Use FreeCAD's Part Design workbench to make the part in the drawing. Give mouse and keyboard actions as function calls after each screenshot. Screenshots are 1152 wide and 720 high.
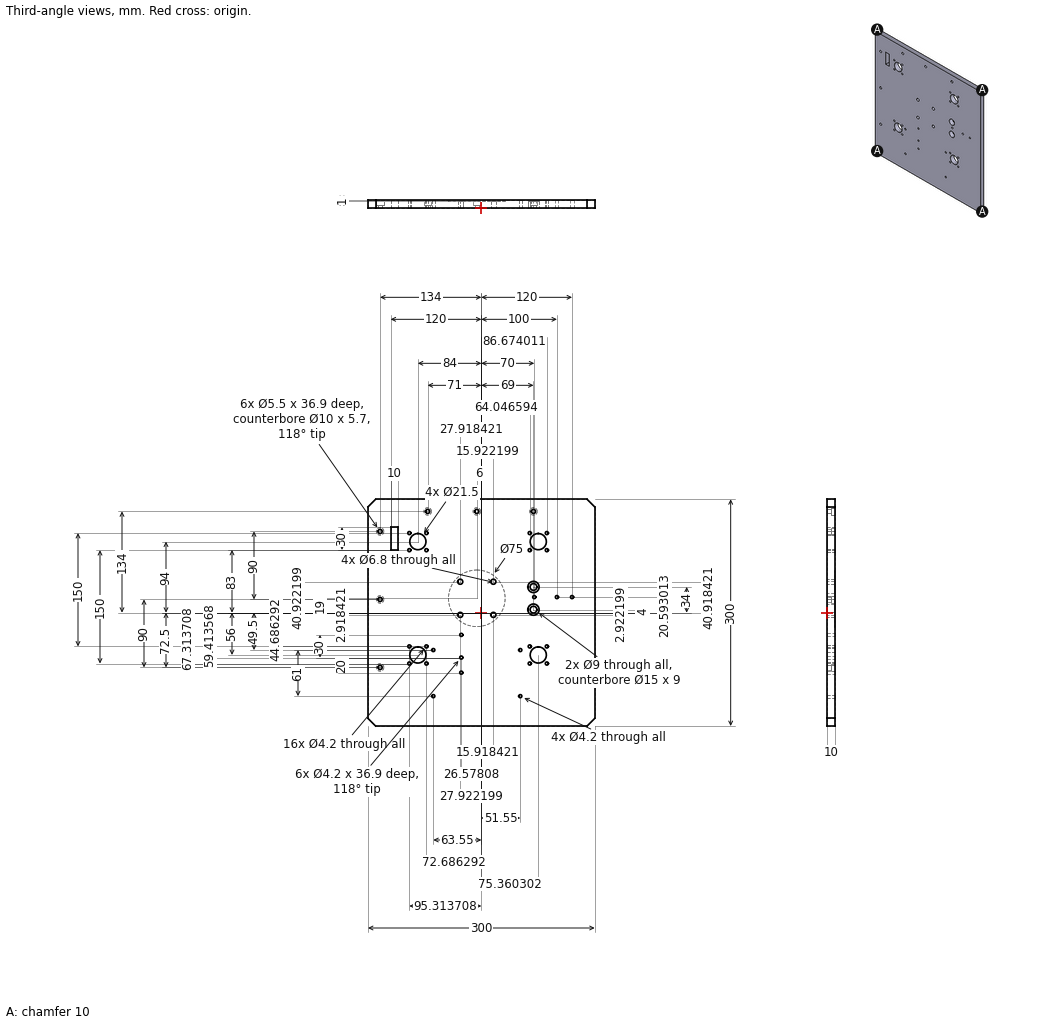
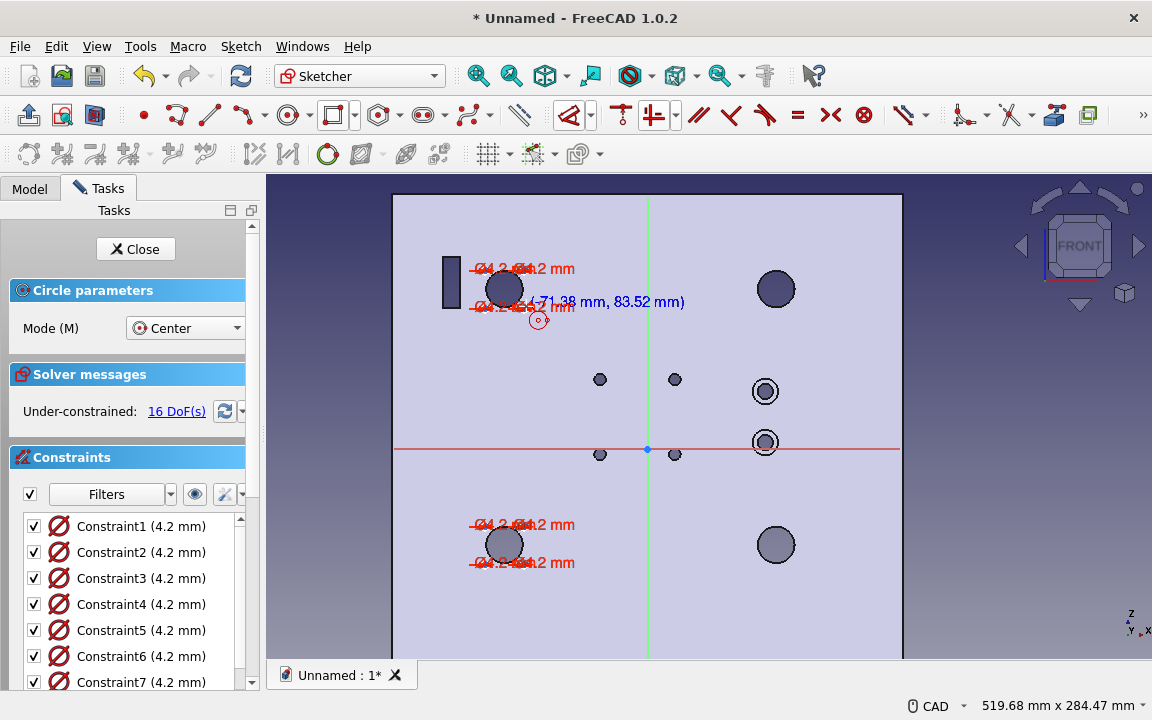
scroll(757, 308, up, 10)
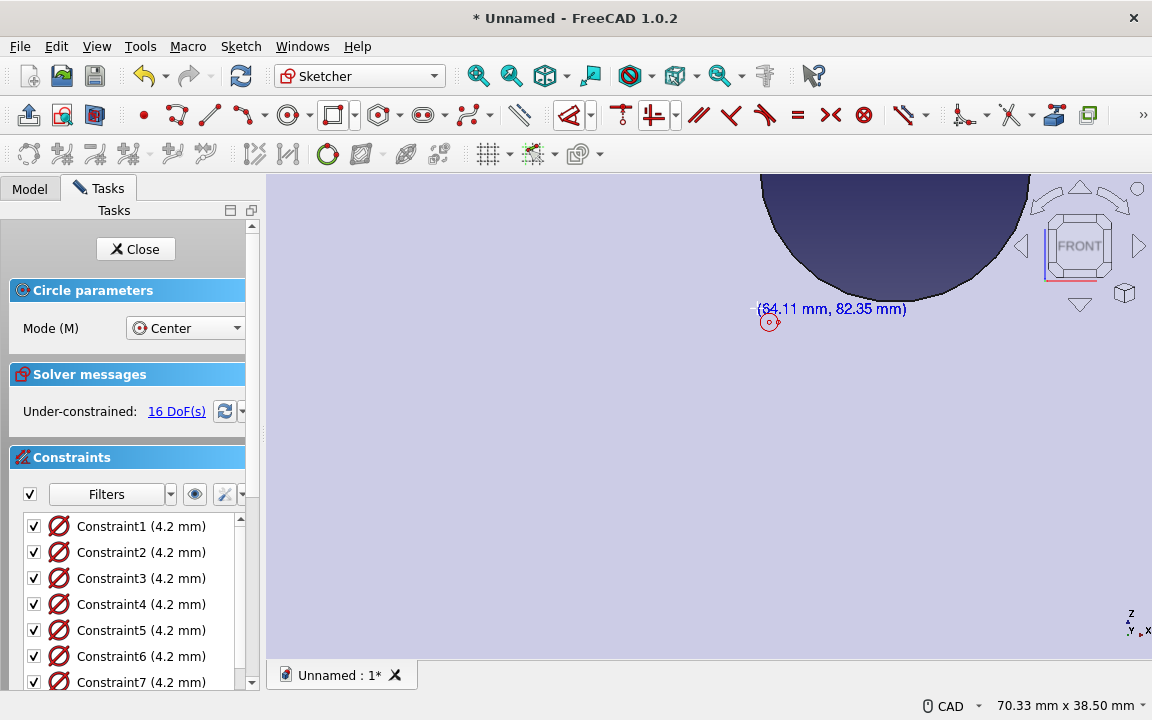
scroll(758, 308, down, 10)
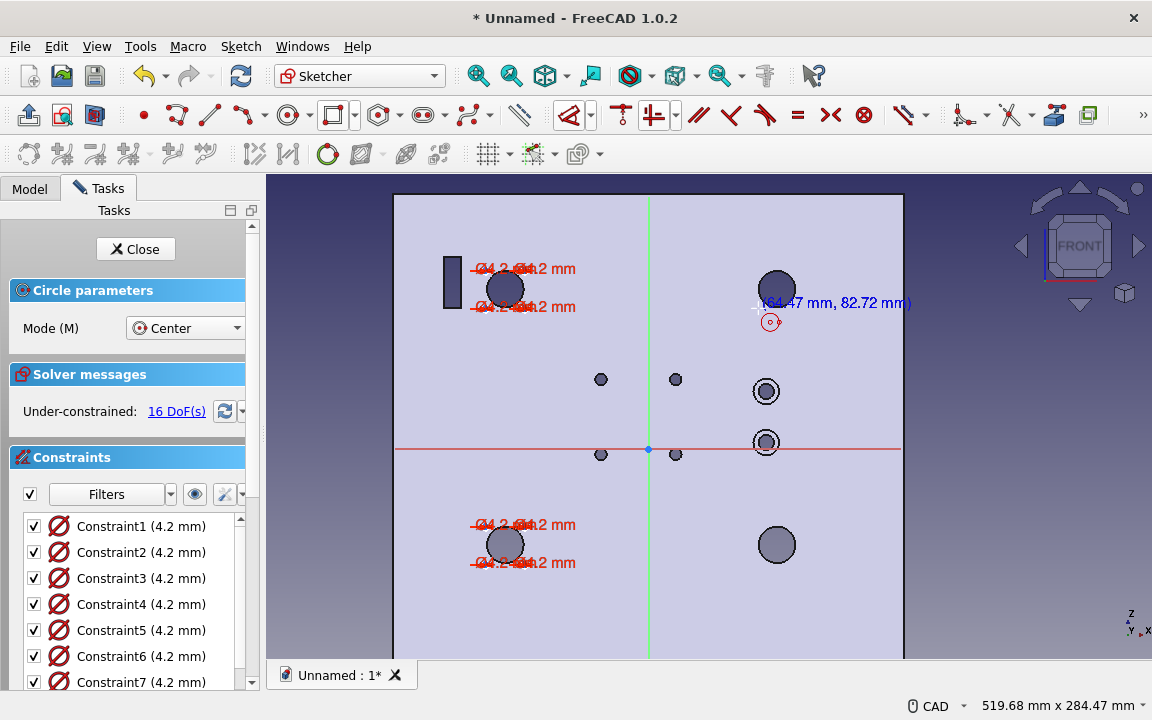
click(758, 308)
move(760, 306)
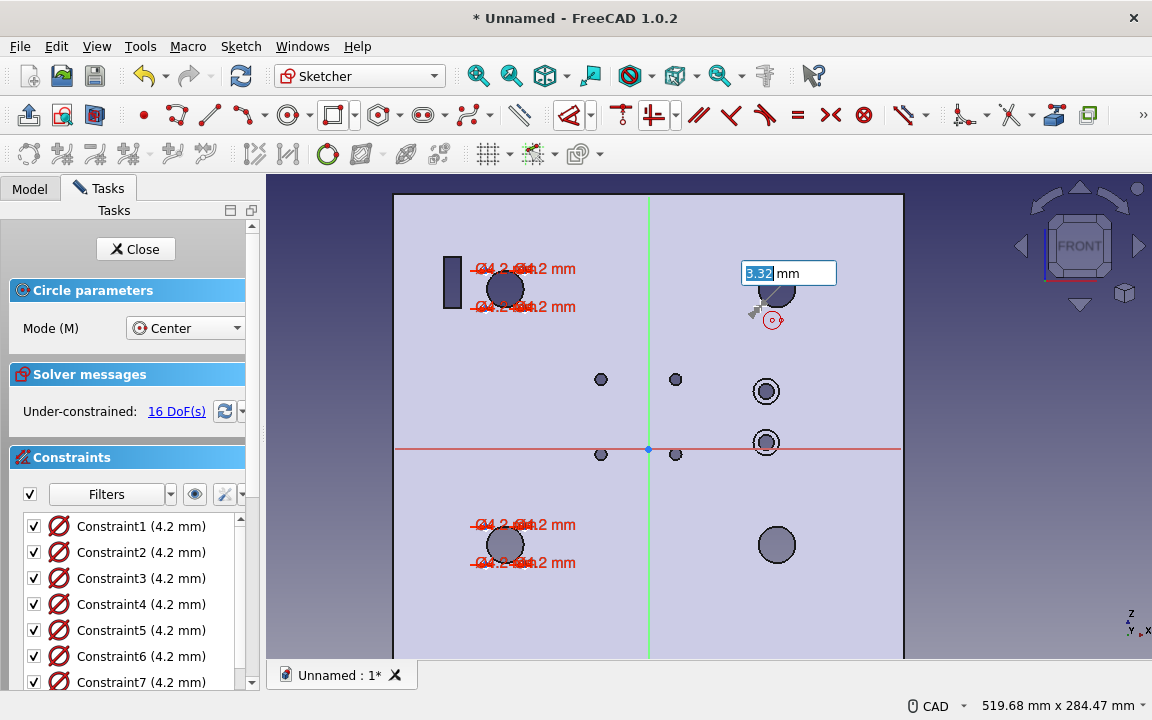
text(4.2)
key(Return)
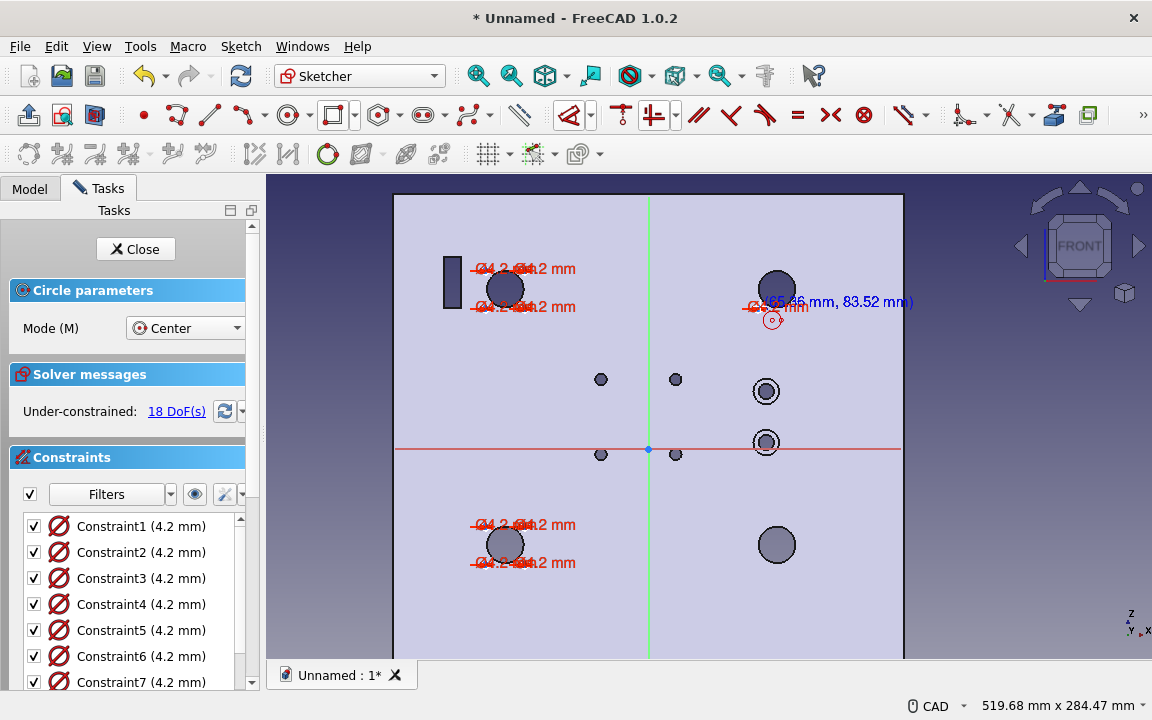
scroll(758, 270, up, 10)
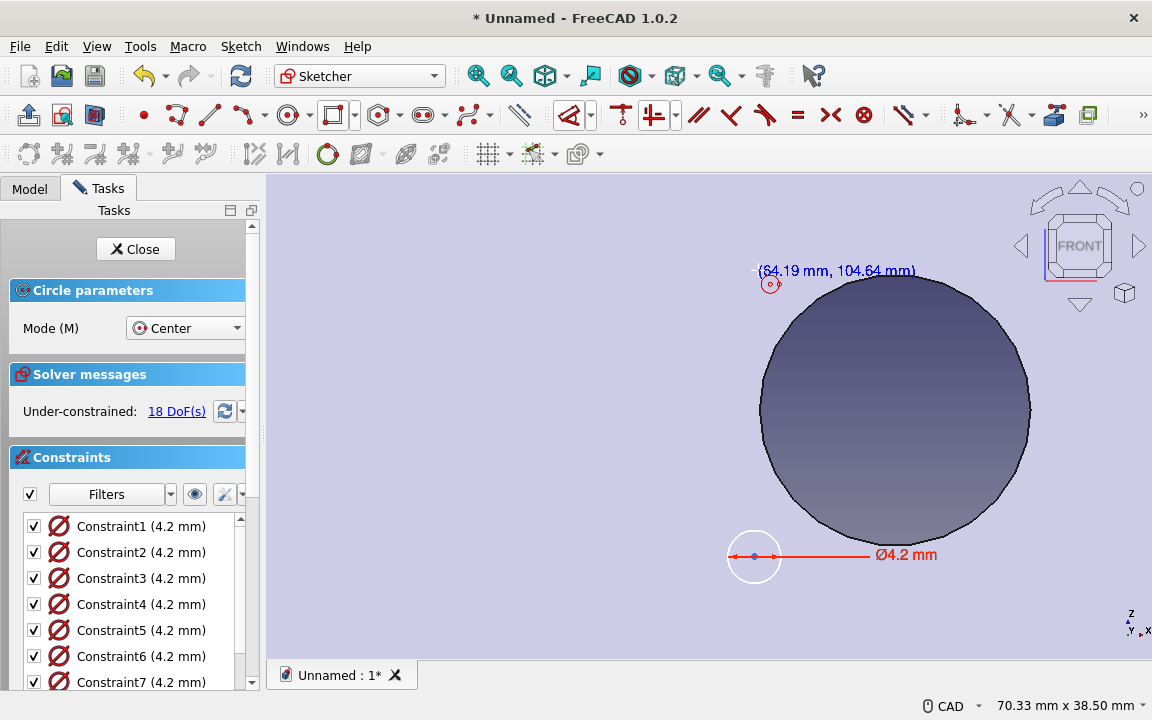
scroll(758, 270, down, 10)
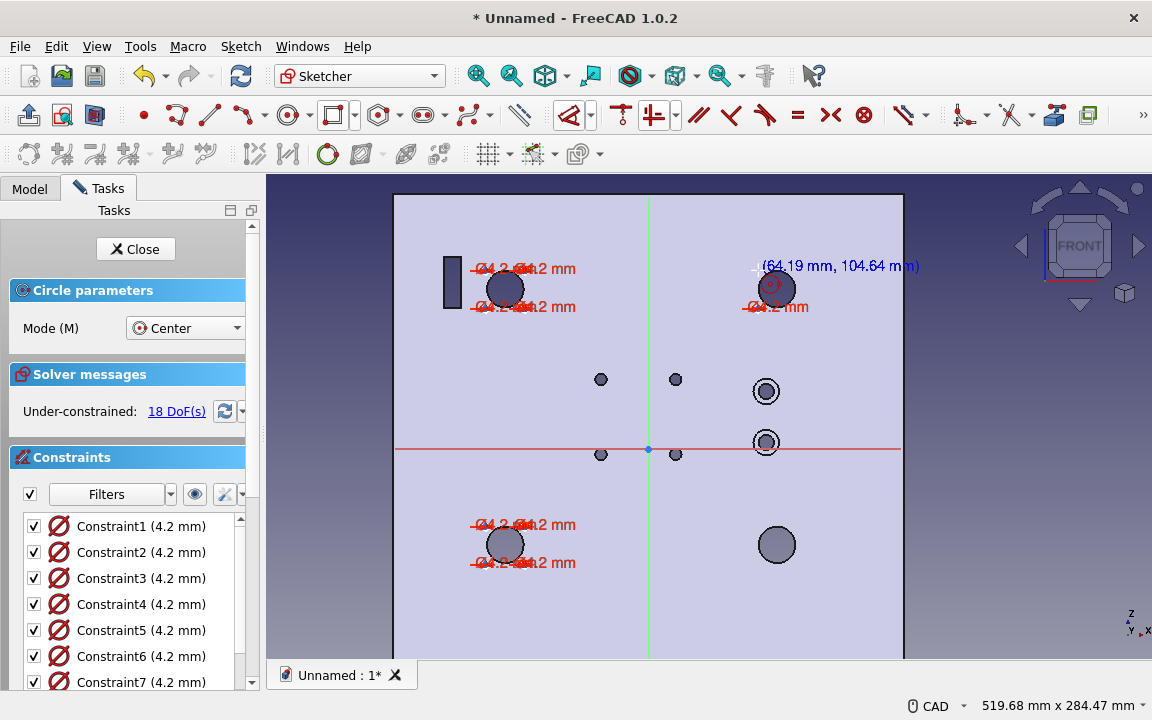
click(758, 270)
move(760, 267)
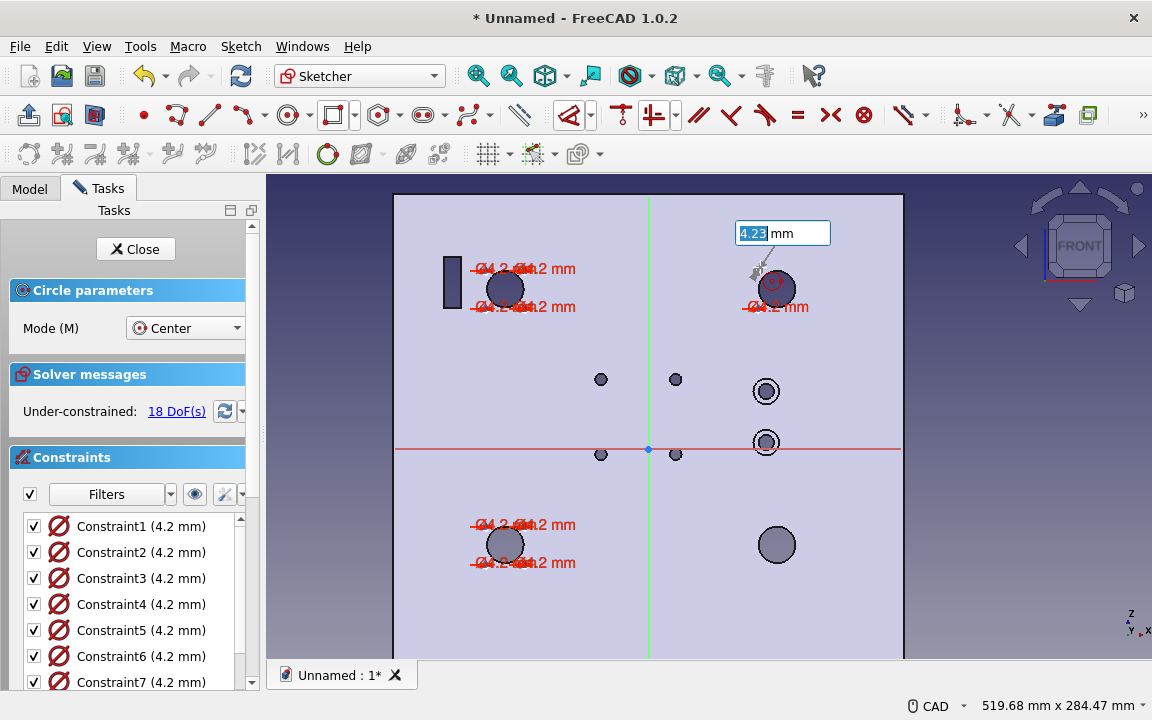
text(4.2)
key(Return)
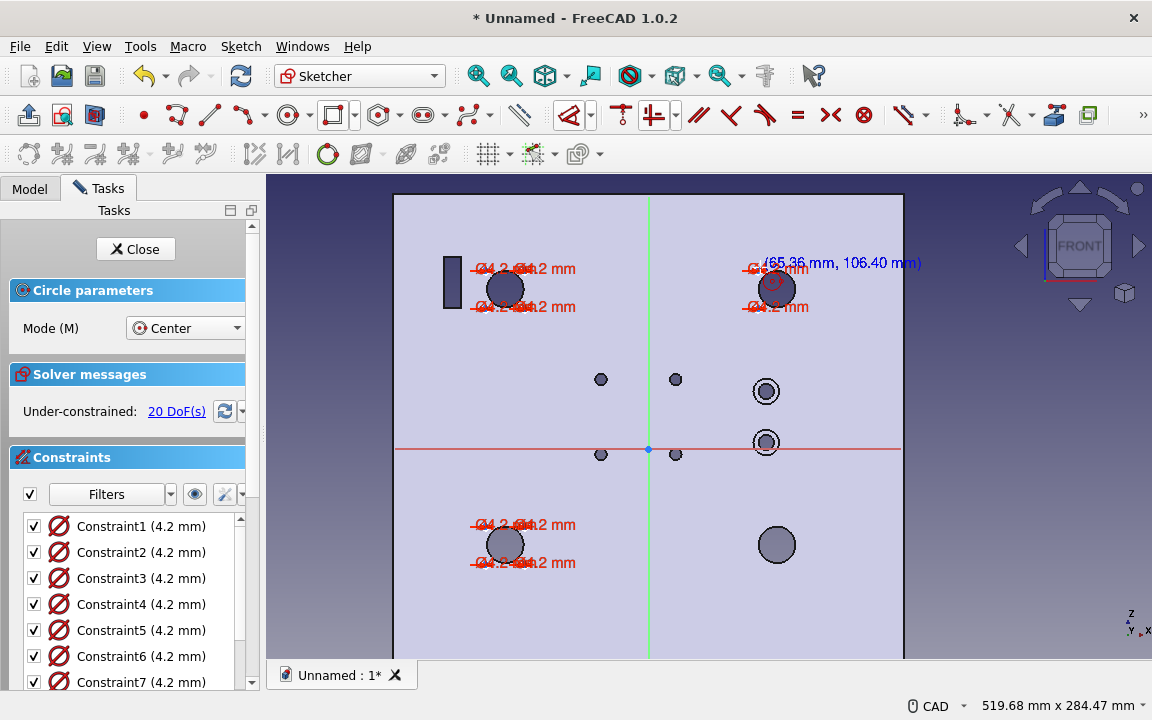
scroll(796, 270, up, 10)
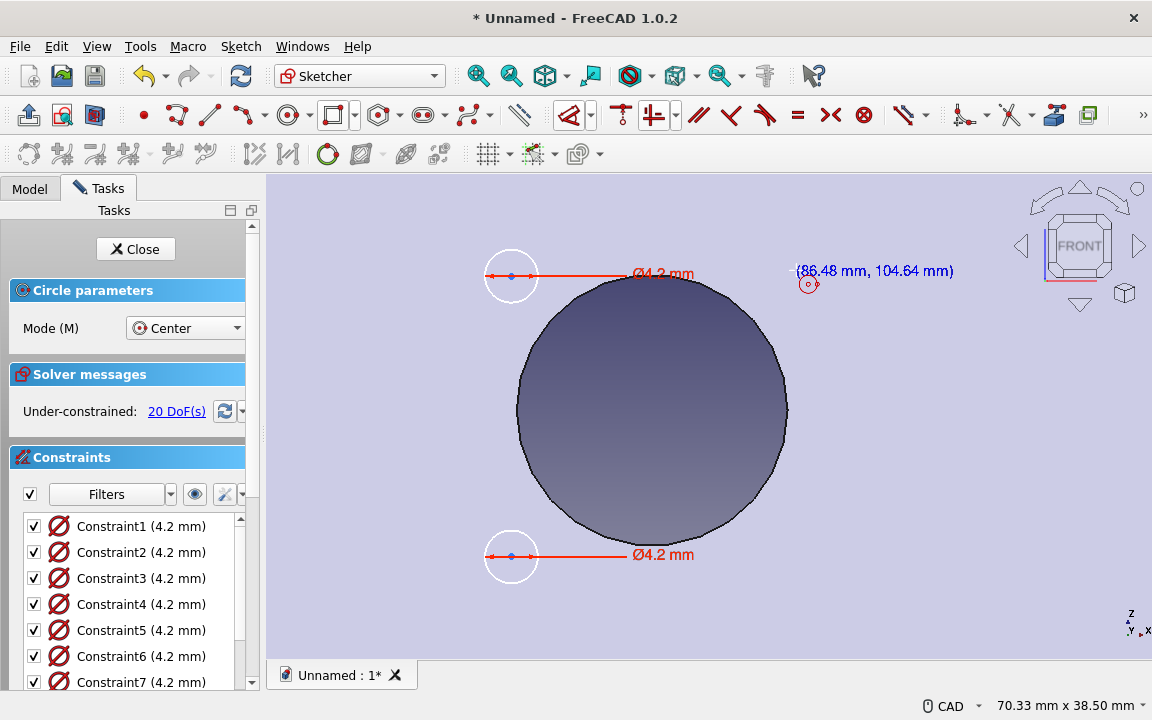
scroll(796, 270, down, 10)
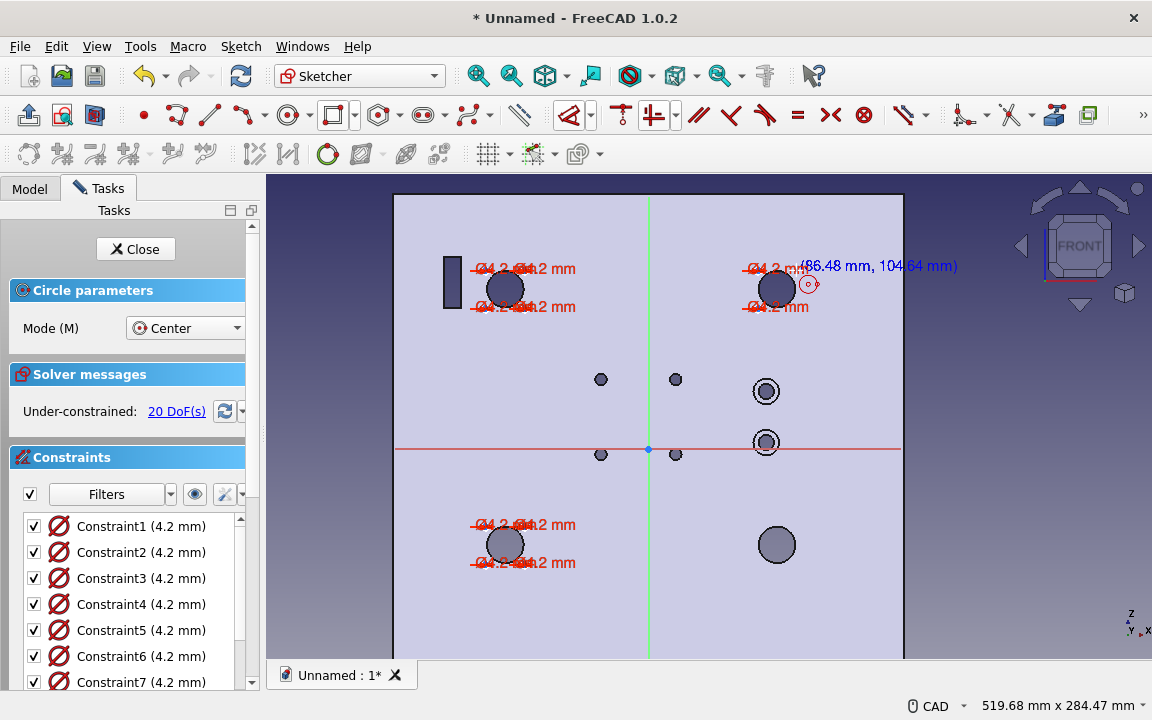
click(796, 270)
move(799, 267)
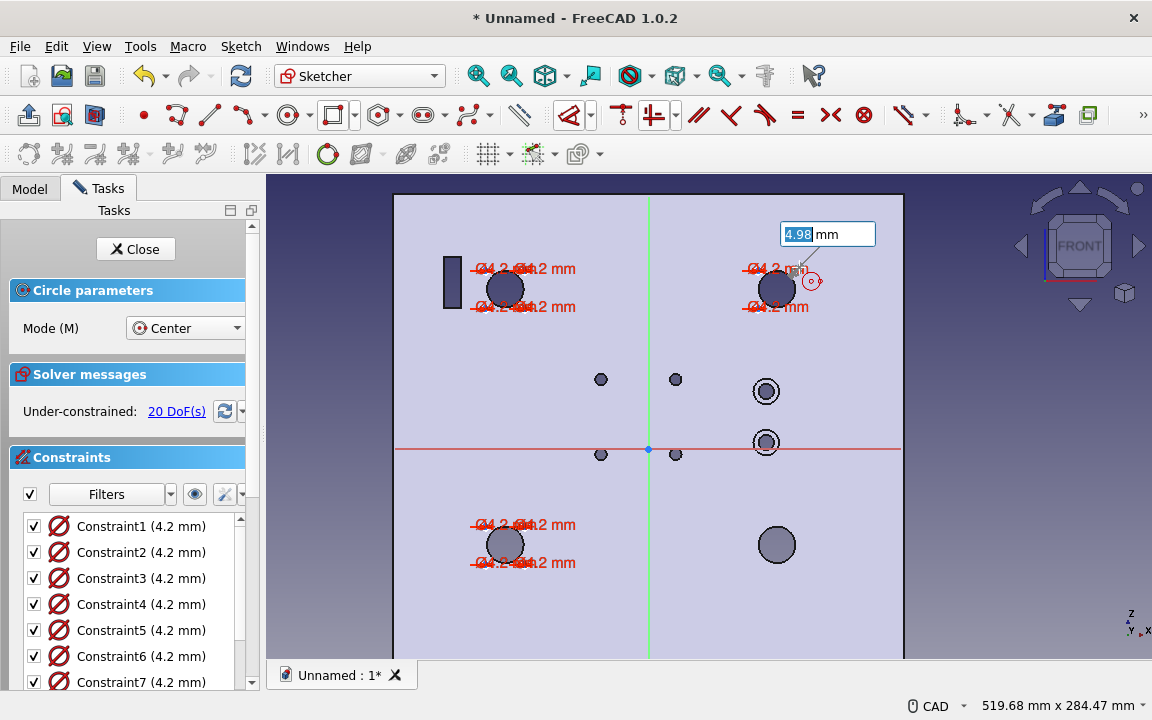
text(4.2)
key(Return)